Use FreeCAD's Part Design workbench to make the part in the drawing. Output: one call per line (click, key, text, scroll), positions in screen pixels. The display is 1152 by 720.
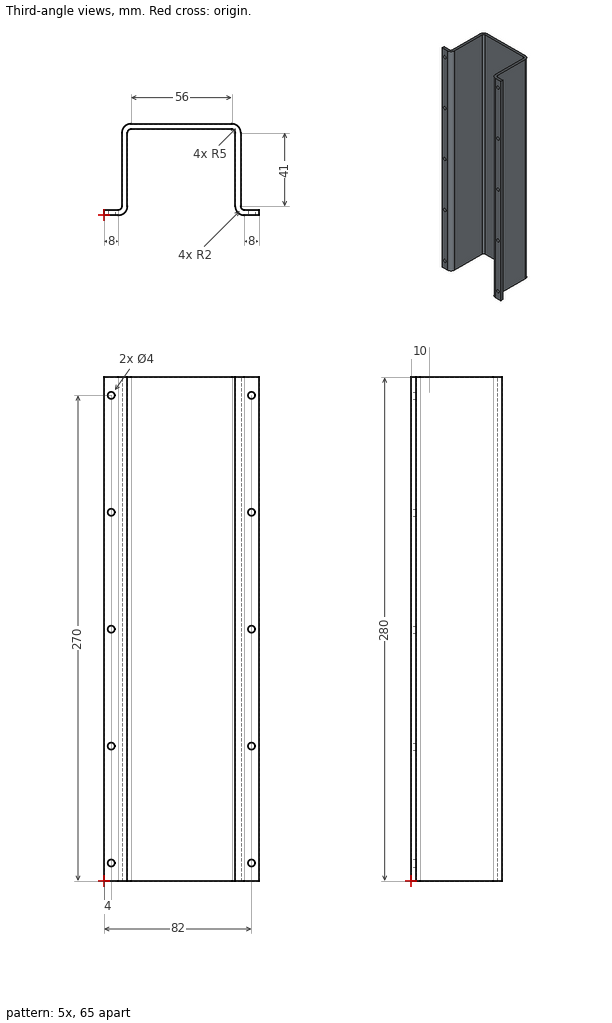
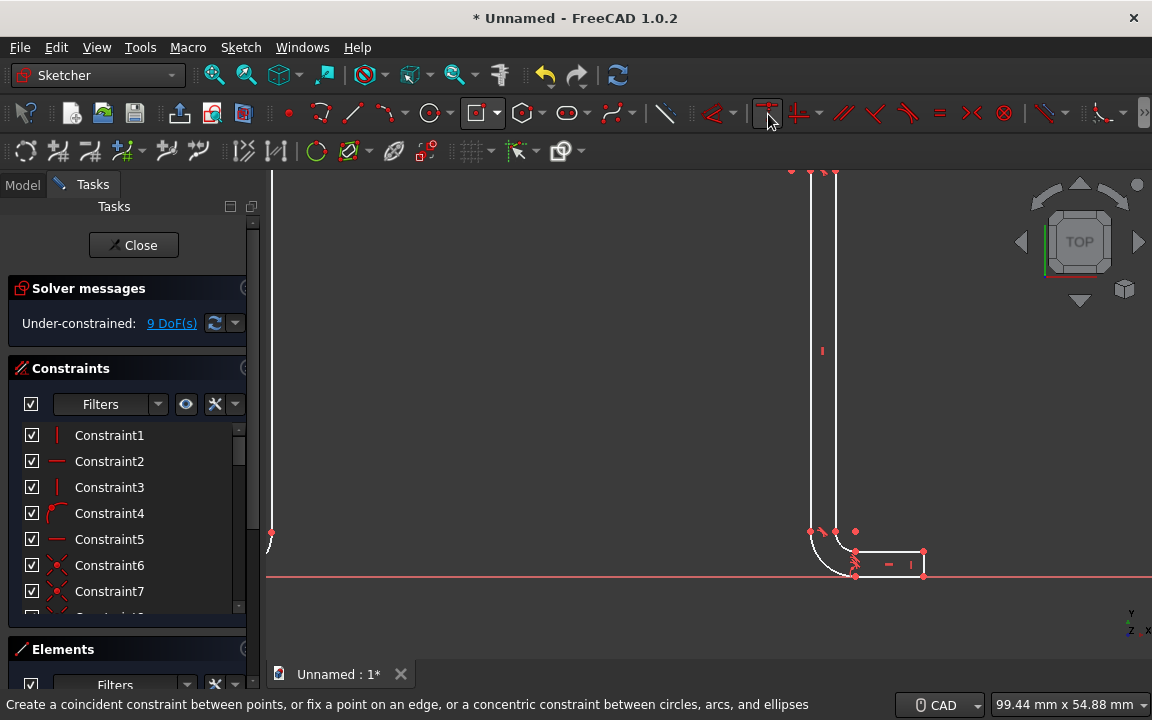
scroll(842, 547, down, 2)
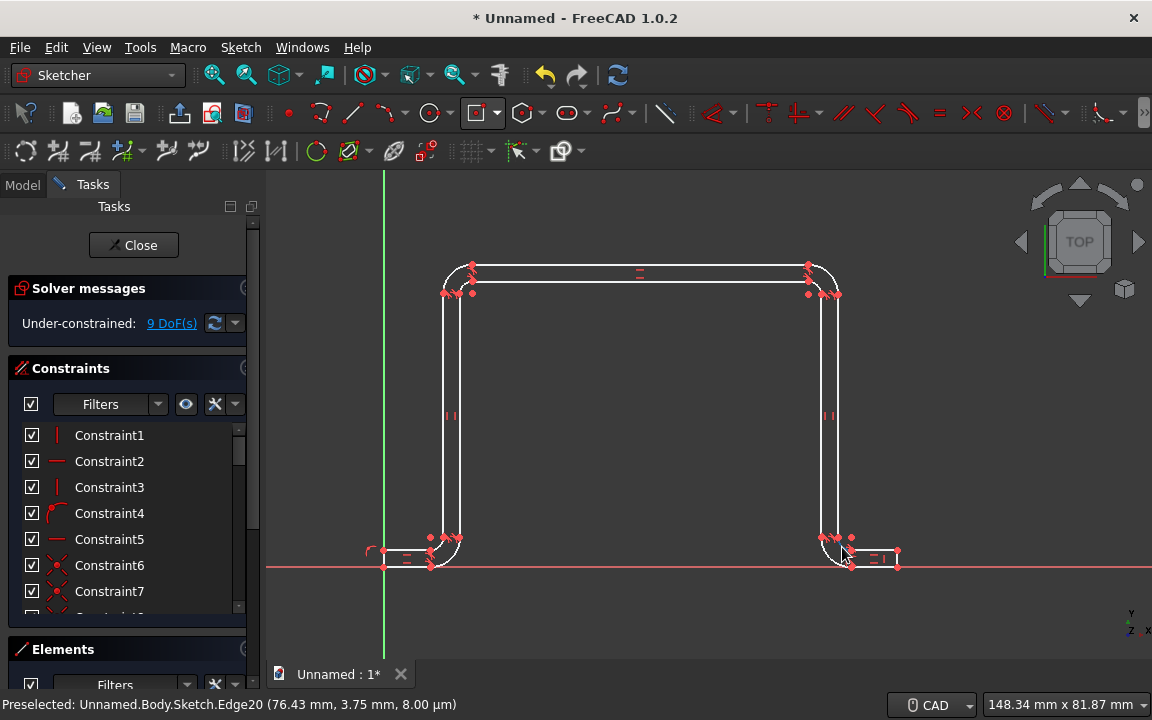
click(835, 281)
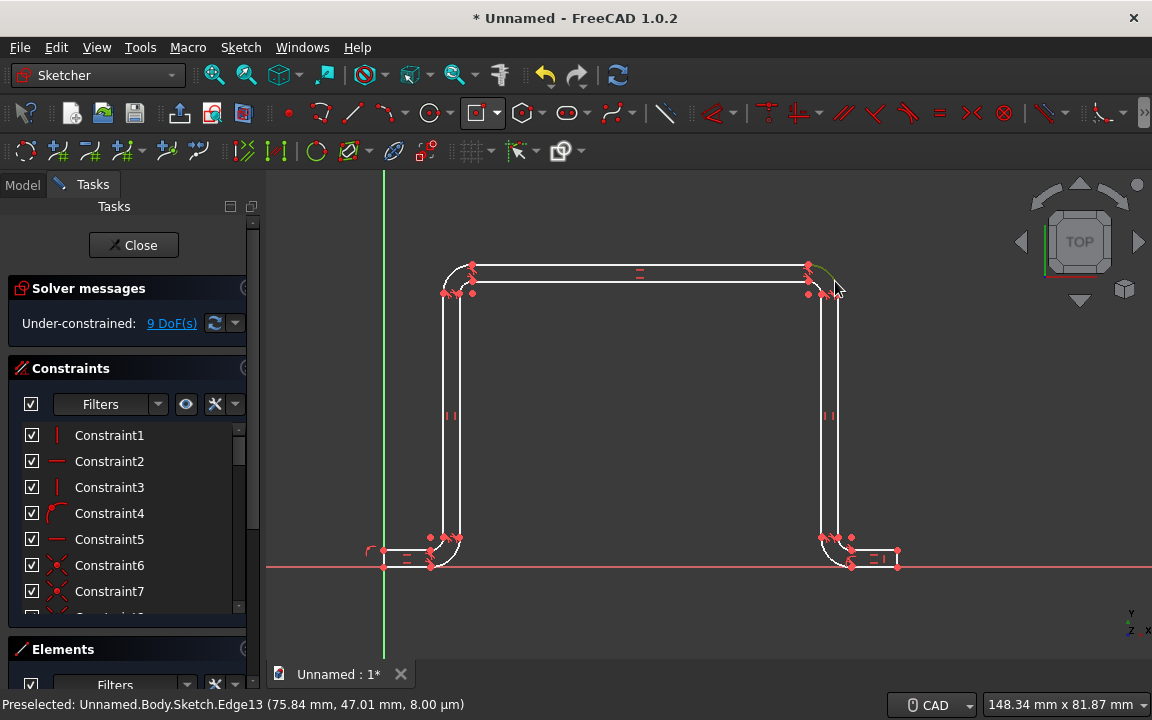
click(459, 268)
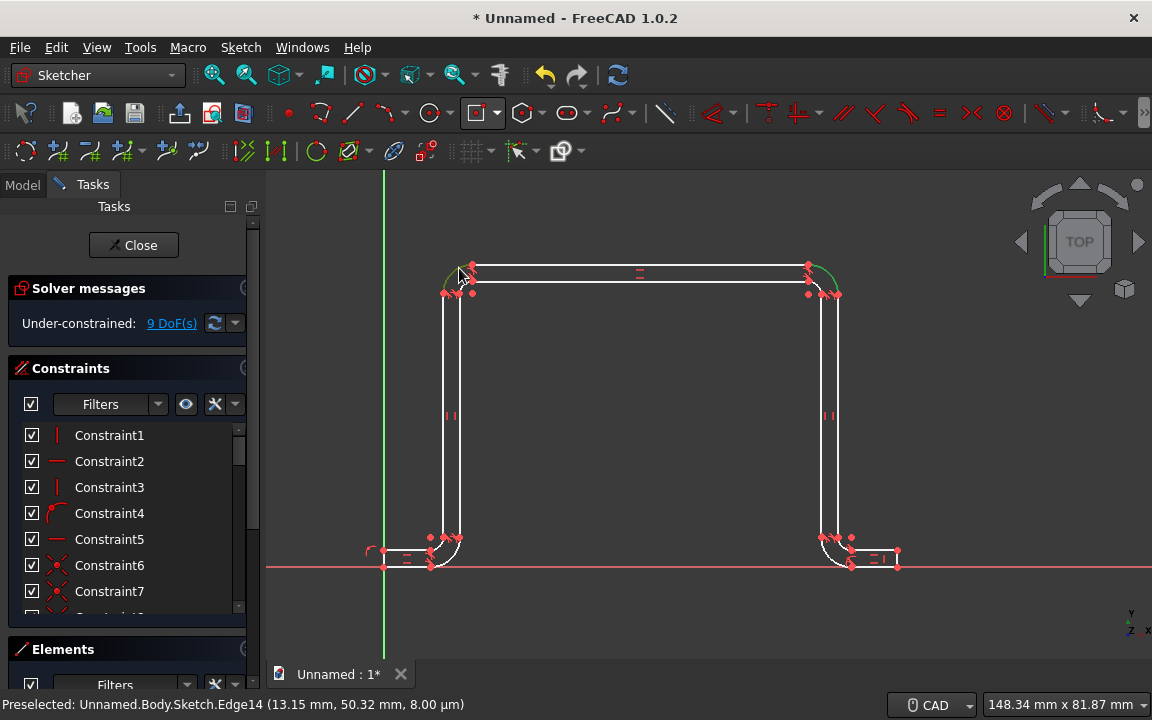
click(444, 564)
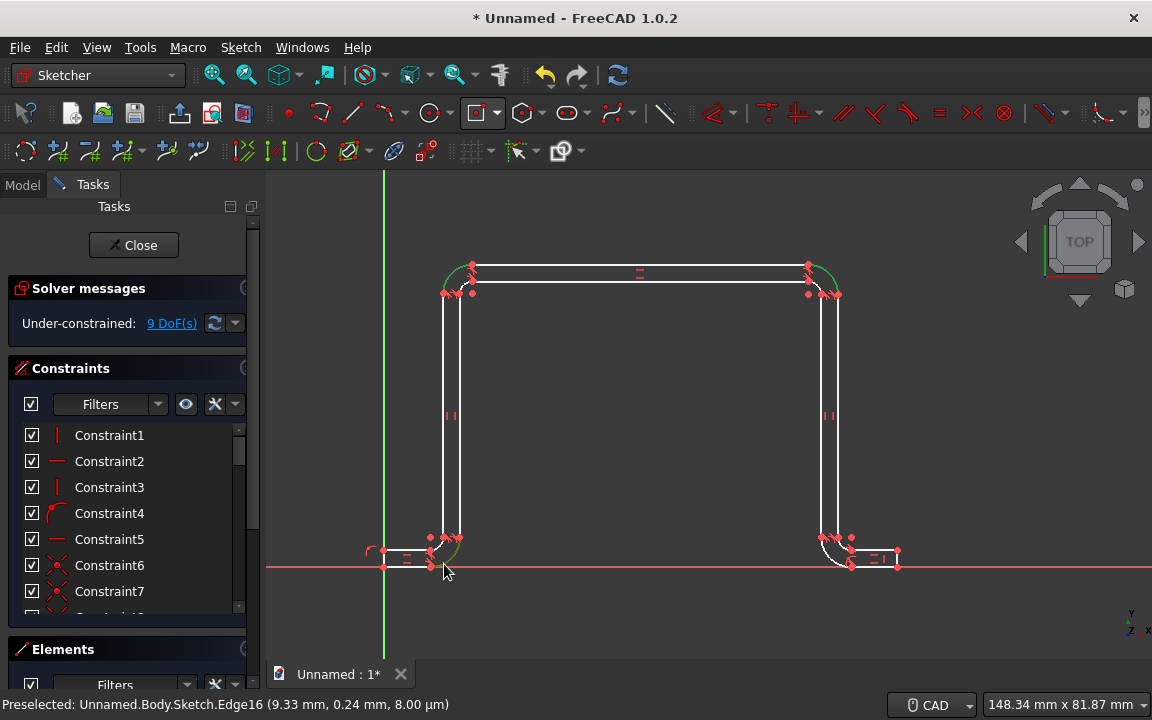
click(825, 551)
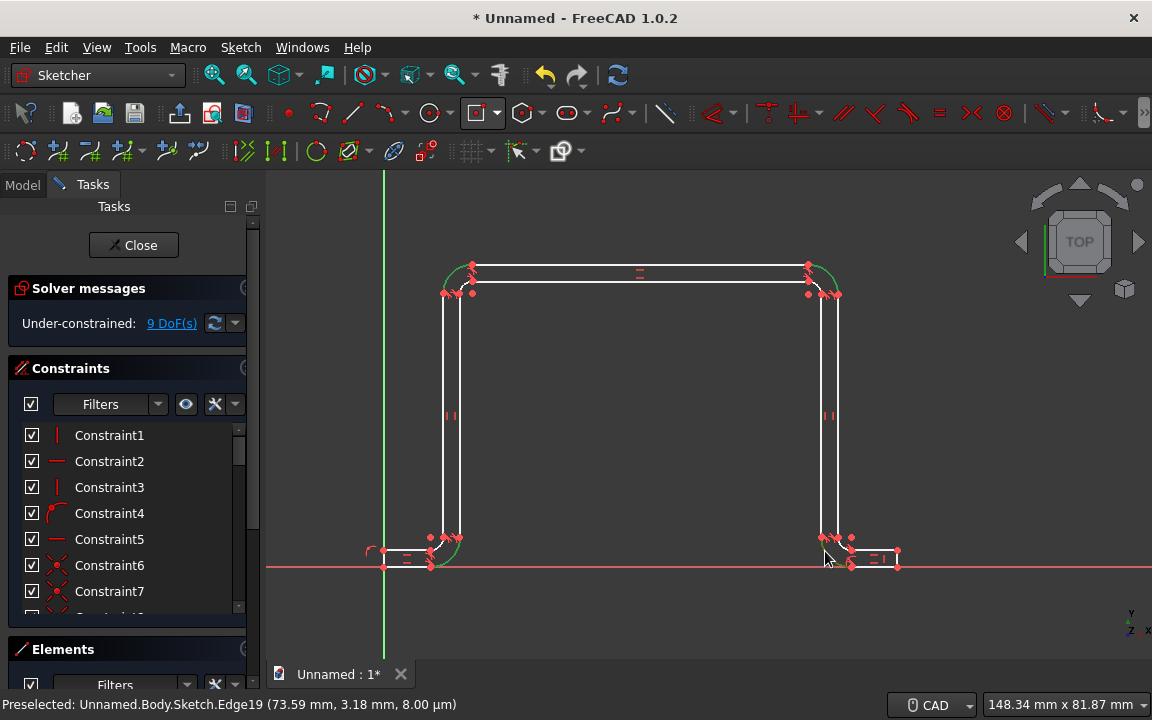
key(e)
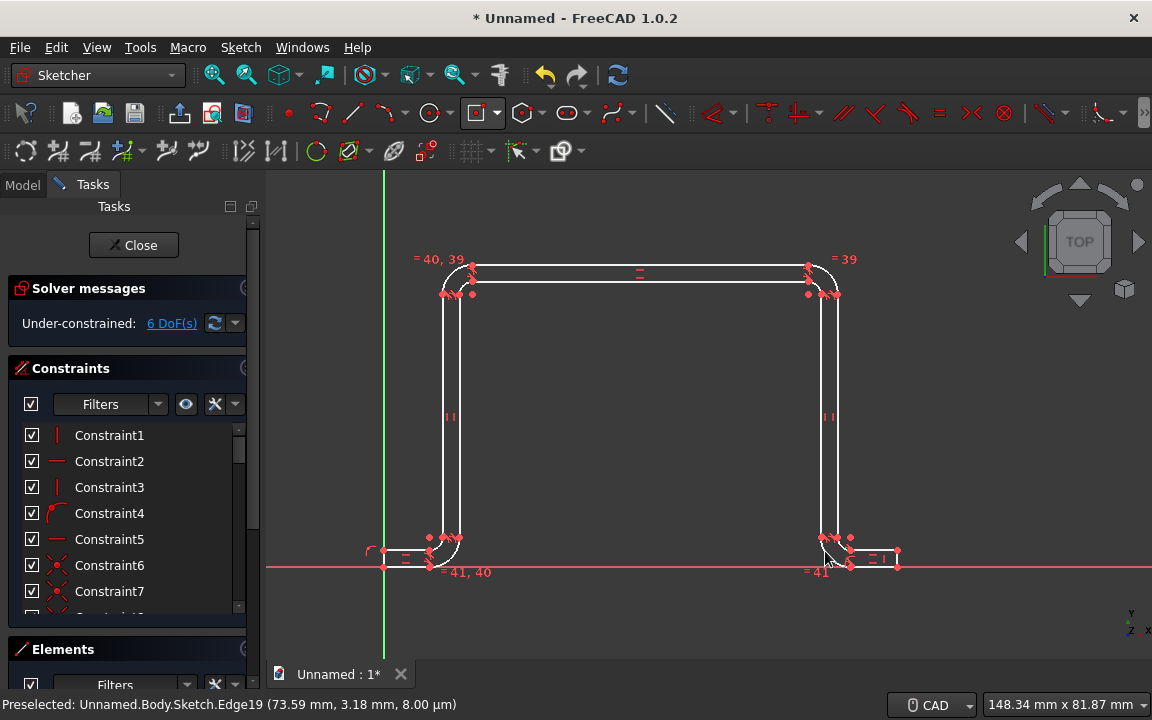
scroll(835, 281, up, 2)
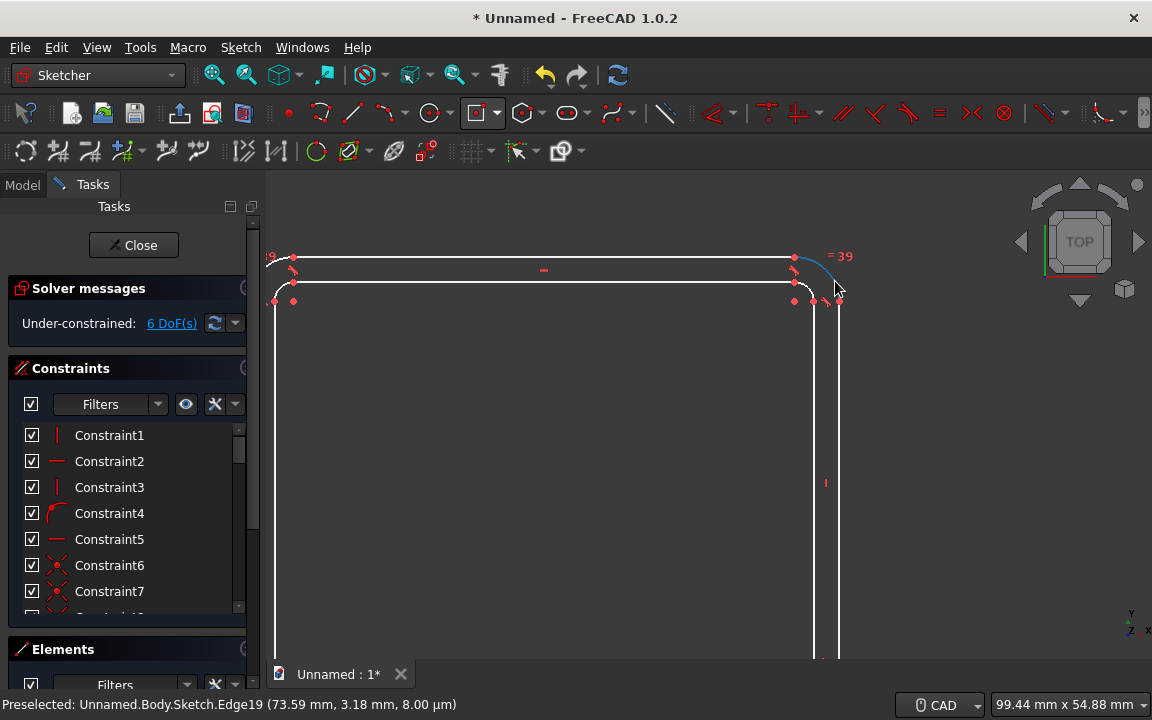
click(834, 281)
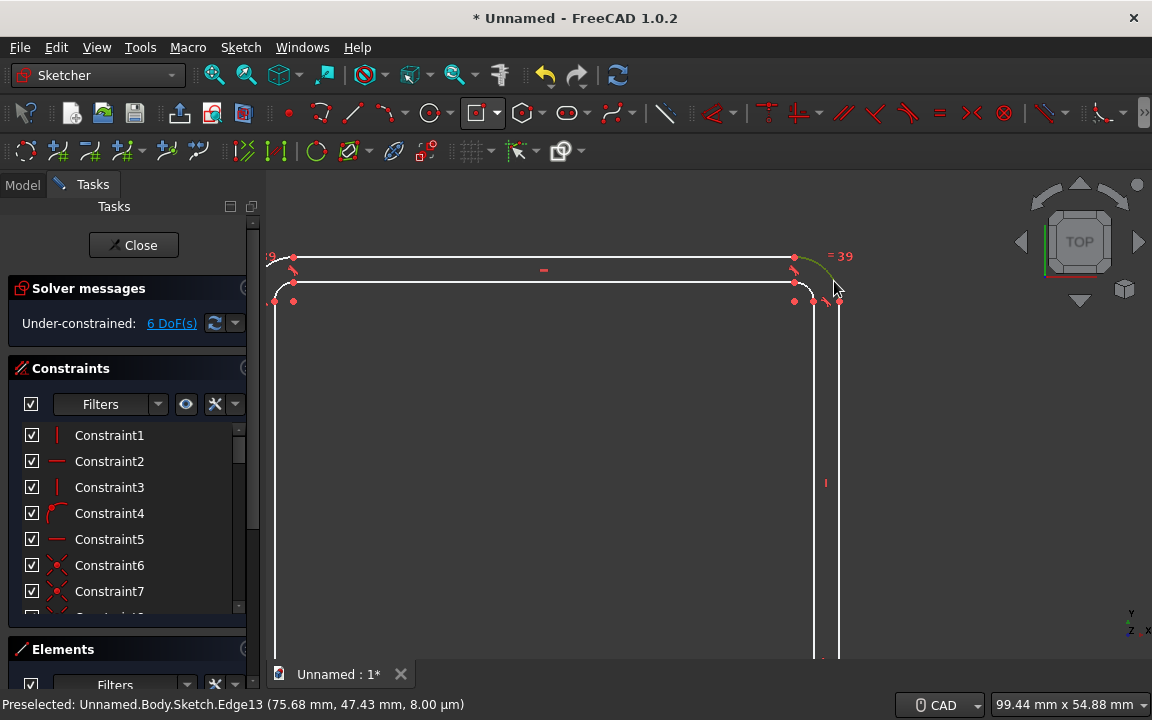
key(k)
key(r)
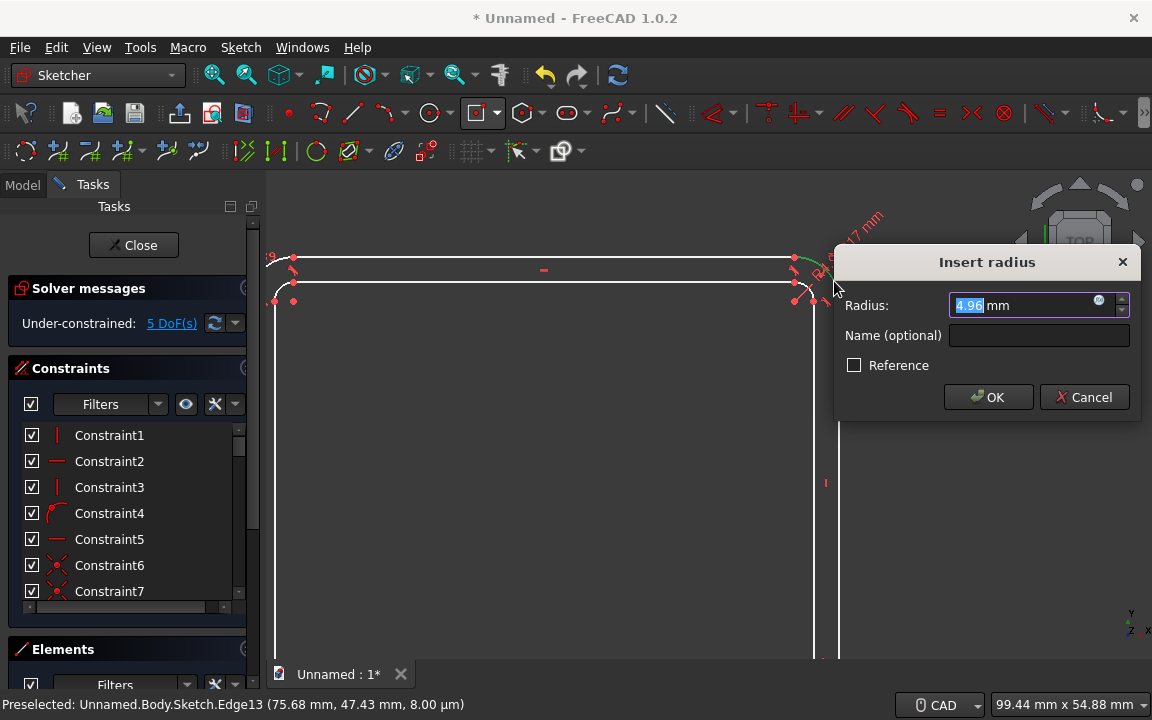
text(5)
key(Return)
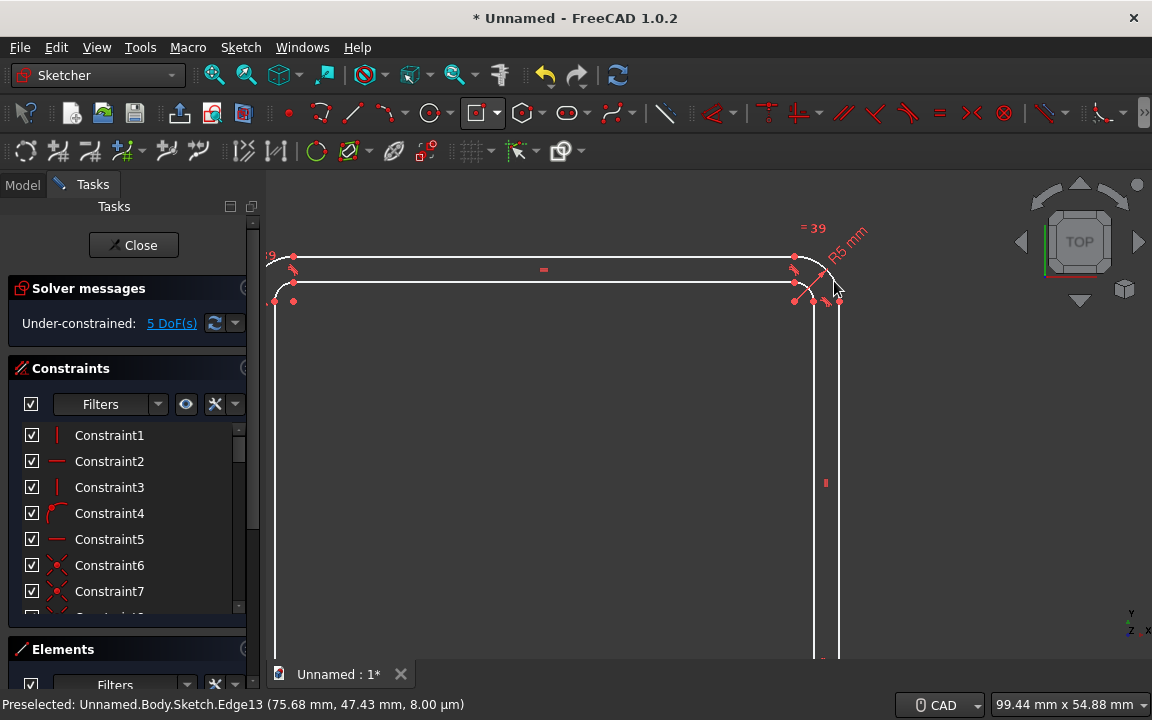
scroll(835, 280, down, 2)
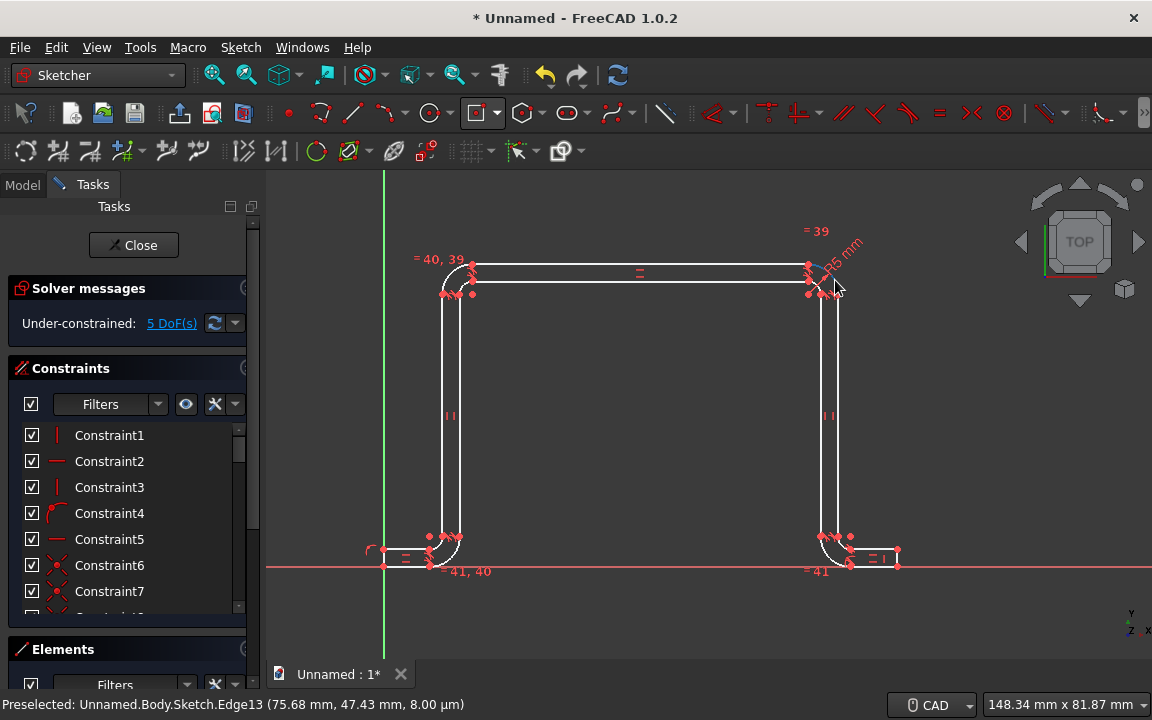
scroll(439, 546, up, 7)